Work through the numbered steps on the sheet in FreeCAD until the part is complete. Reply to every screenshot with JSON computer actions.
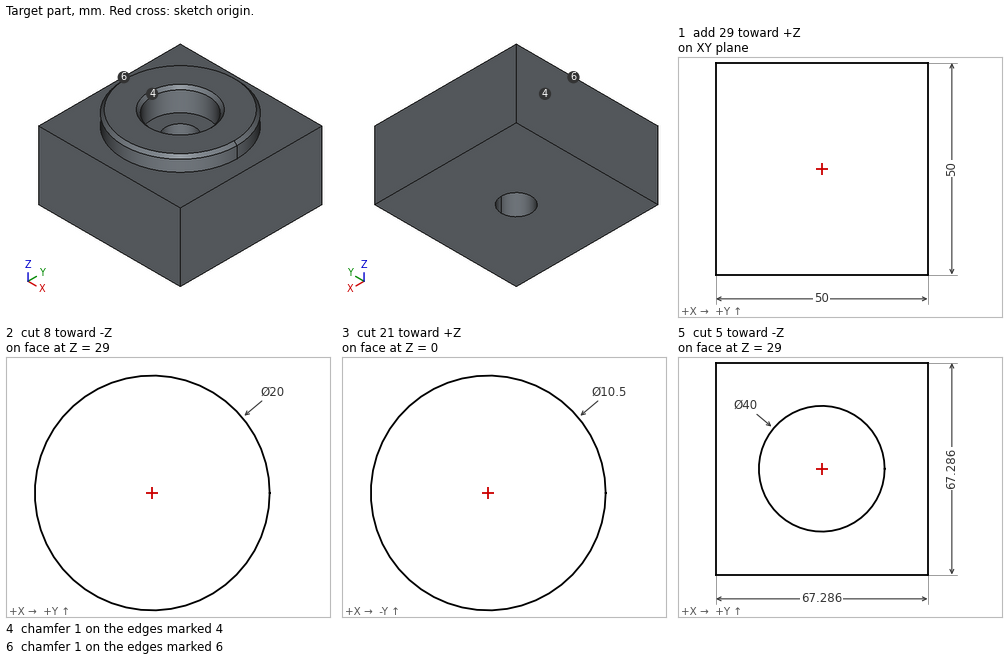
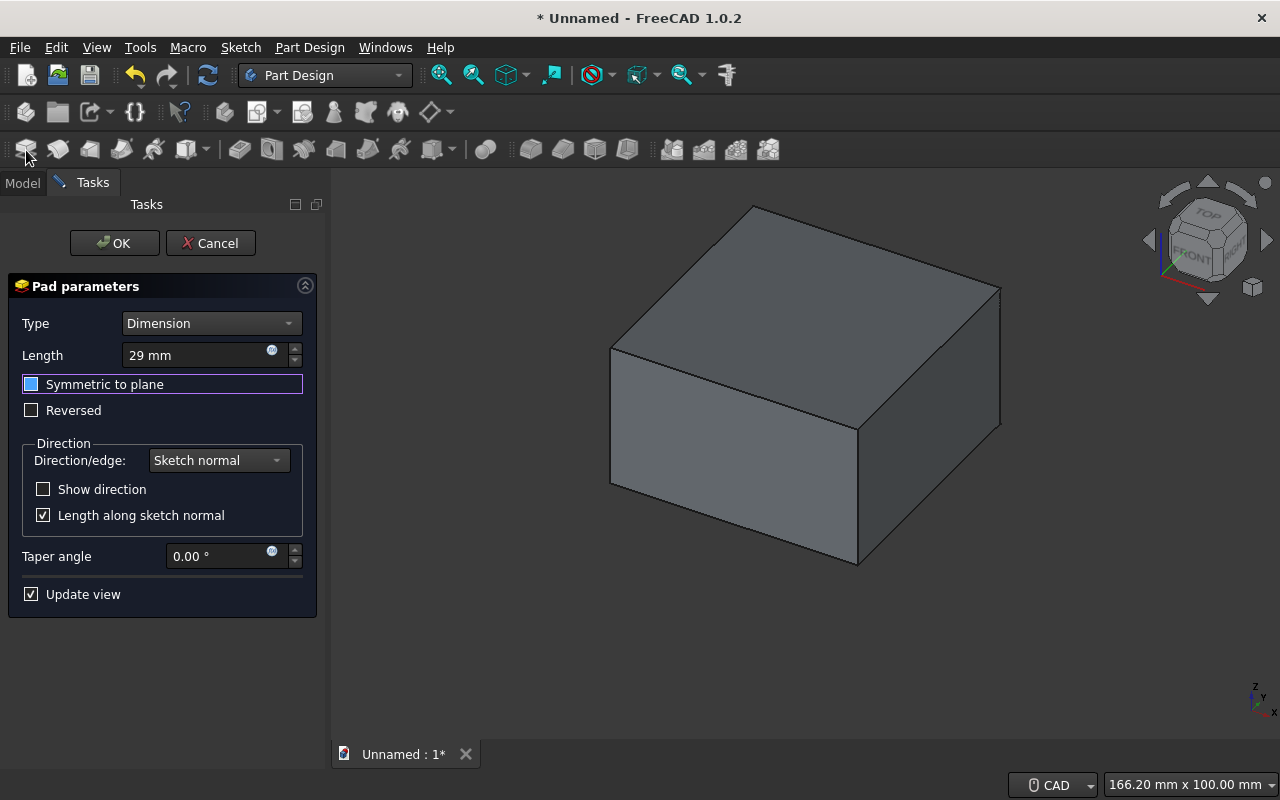
{"action": "left_click", "coordinate": [115, 243]}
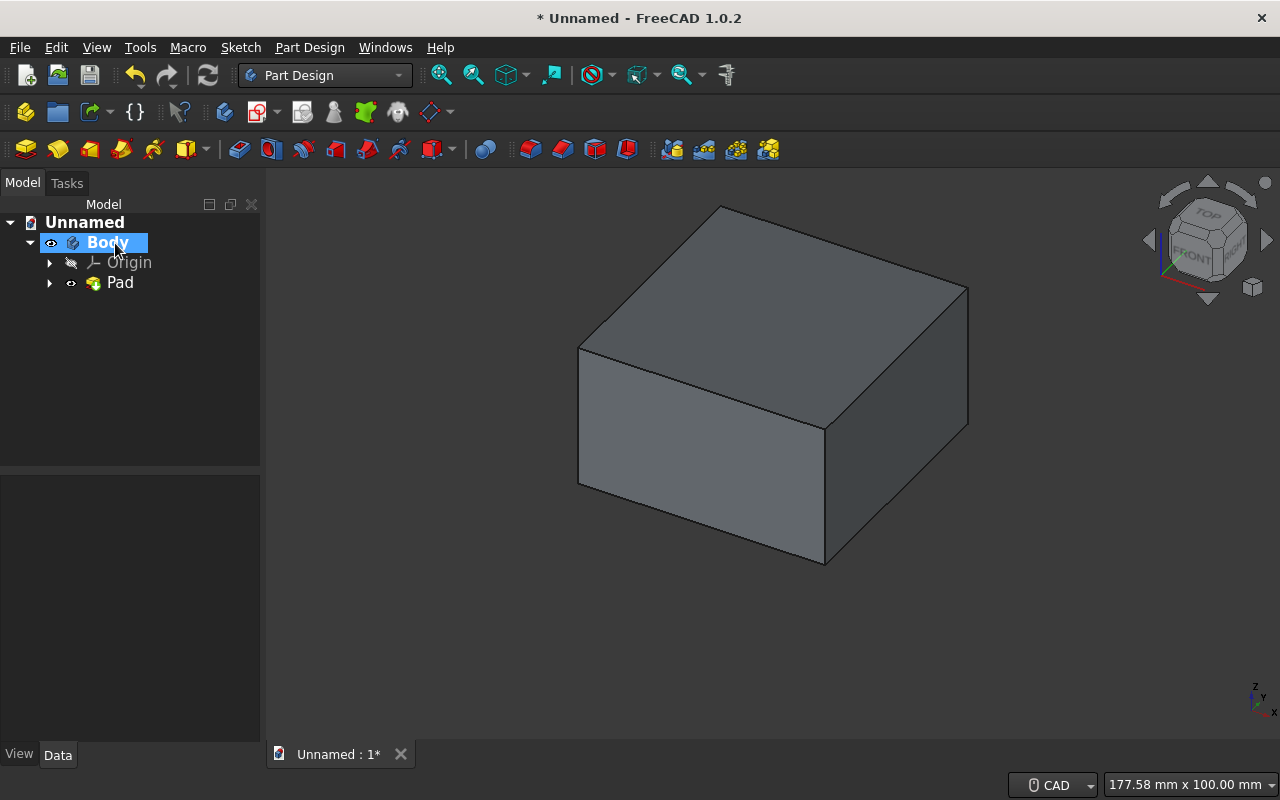
{"action": "left_click", "coordinate": [773, 317]}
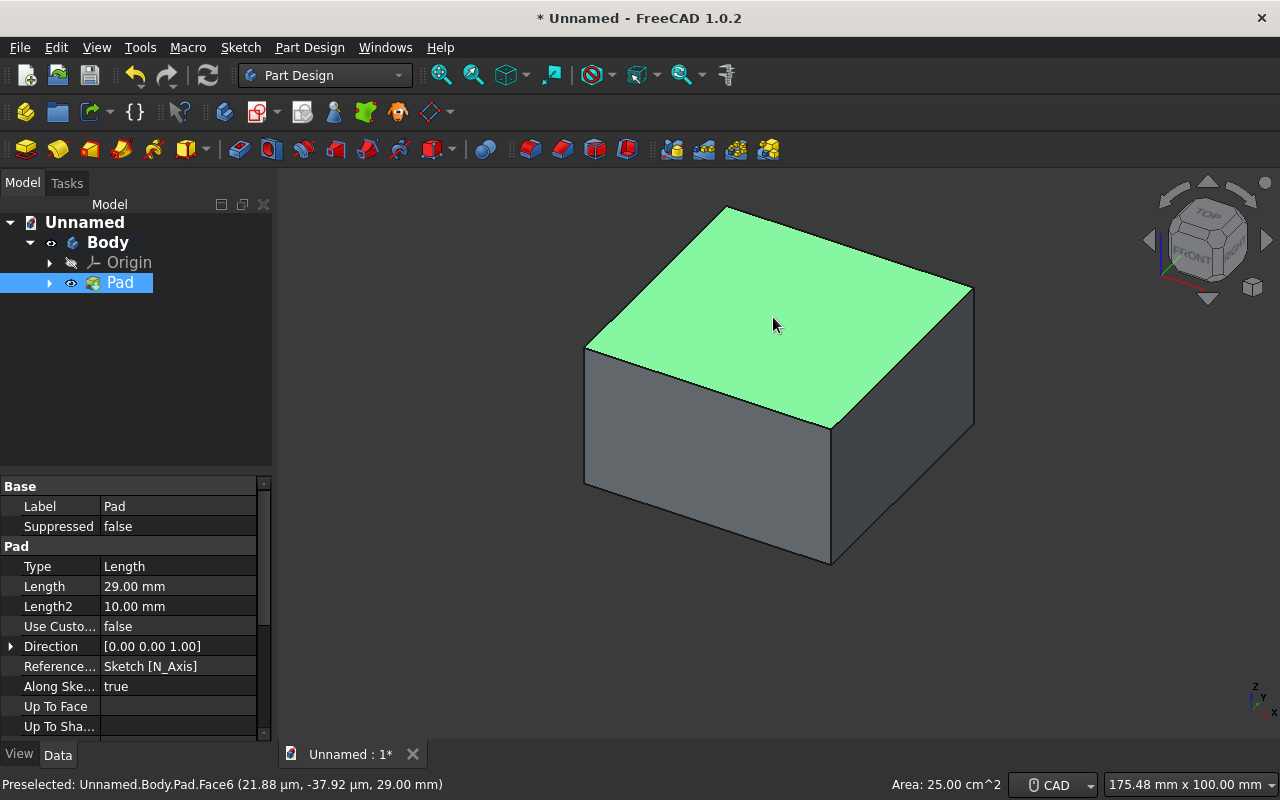
{"action": "left_click", "coordinate": [258, 112]}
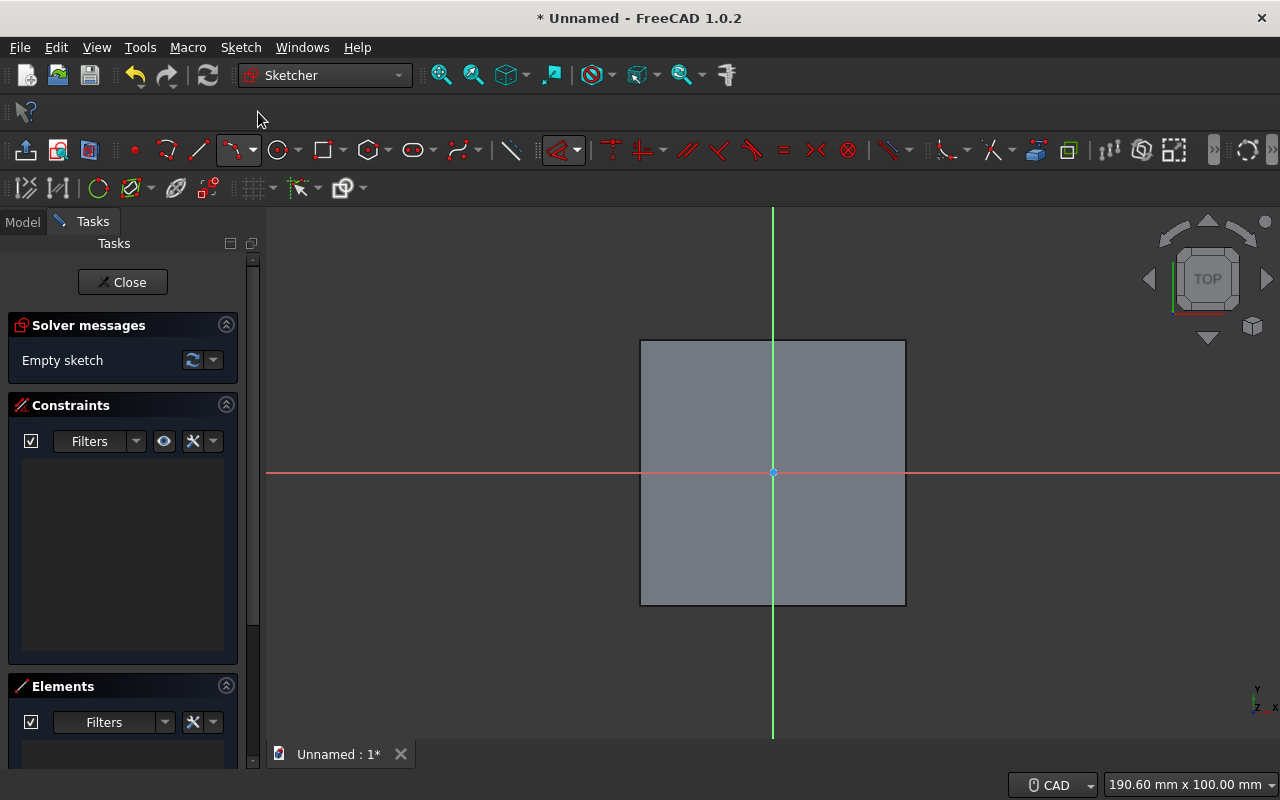
{"action": "scroll", "coordinate": [803, 473], "scroll_direction": "up", "scroll_amount": 6}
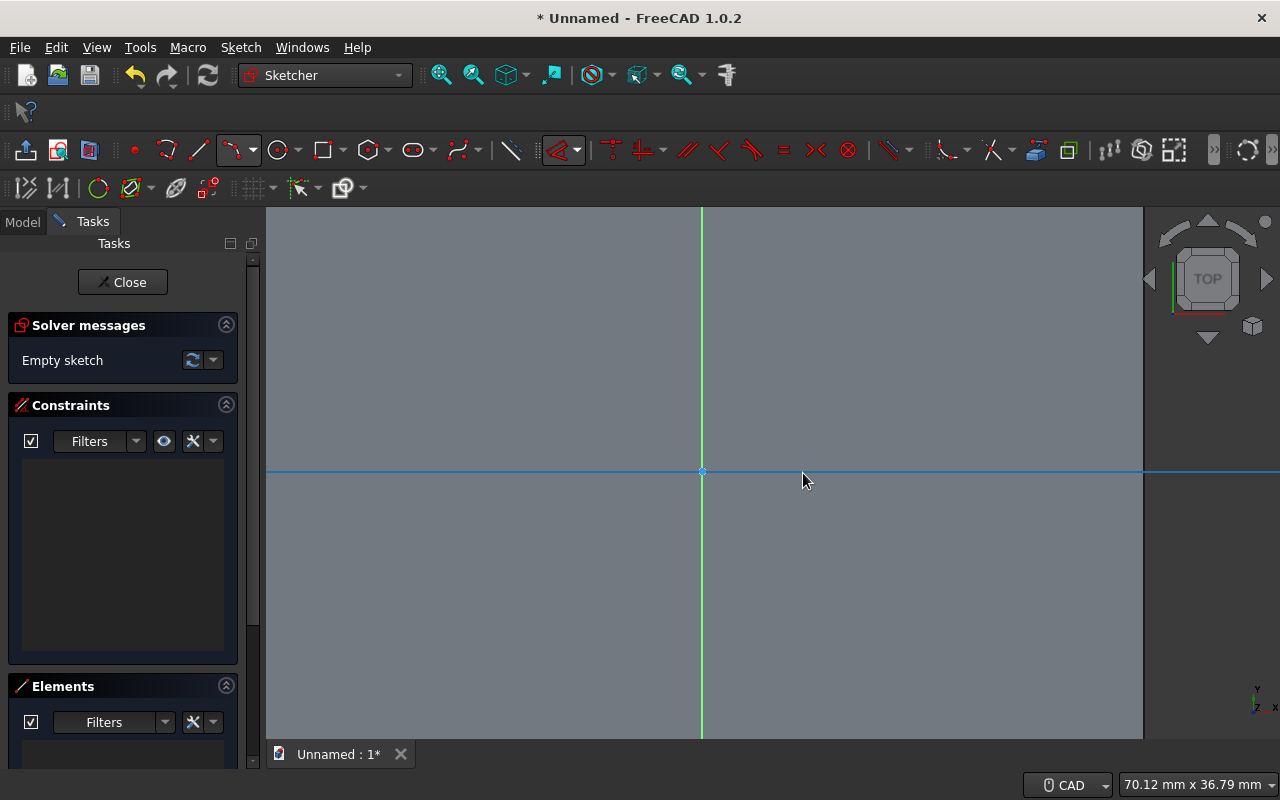
{"action": "left_click", "coordinate": [278, 150]}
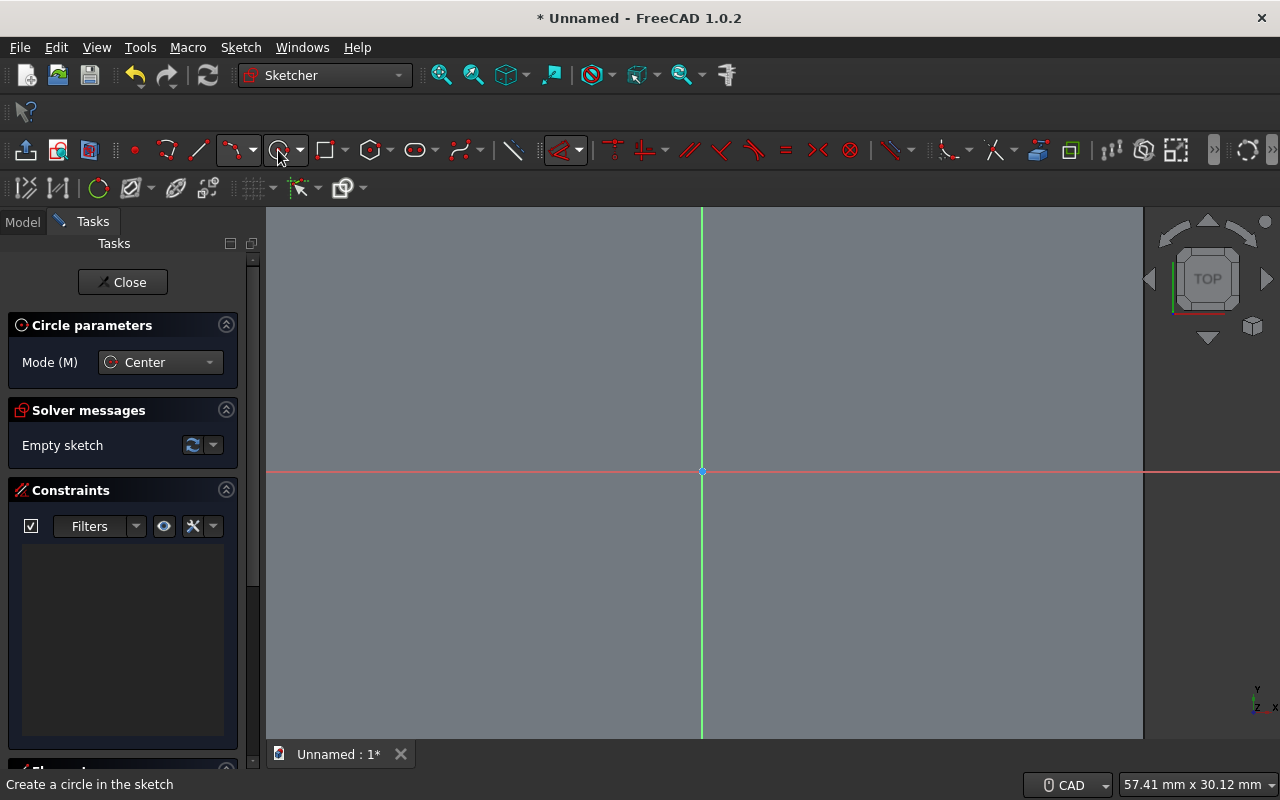
{"action": "left_click", "coordinate": [702, 472]}
{"action": "mouse_move", "coordinate": [827, 347]}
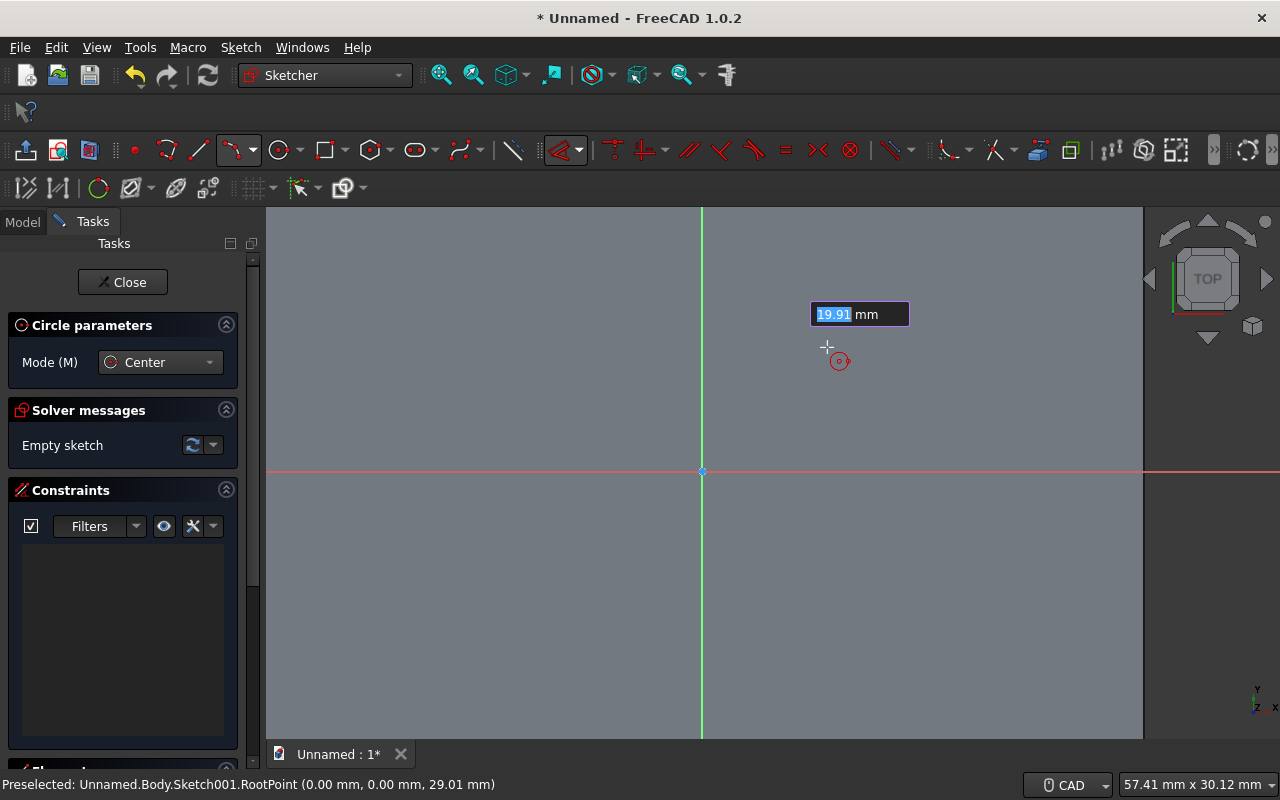
{"action": "type", "text": "20"}
{"action": "key", "text": "Return"}
{"action": "key", "text": "Escape"}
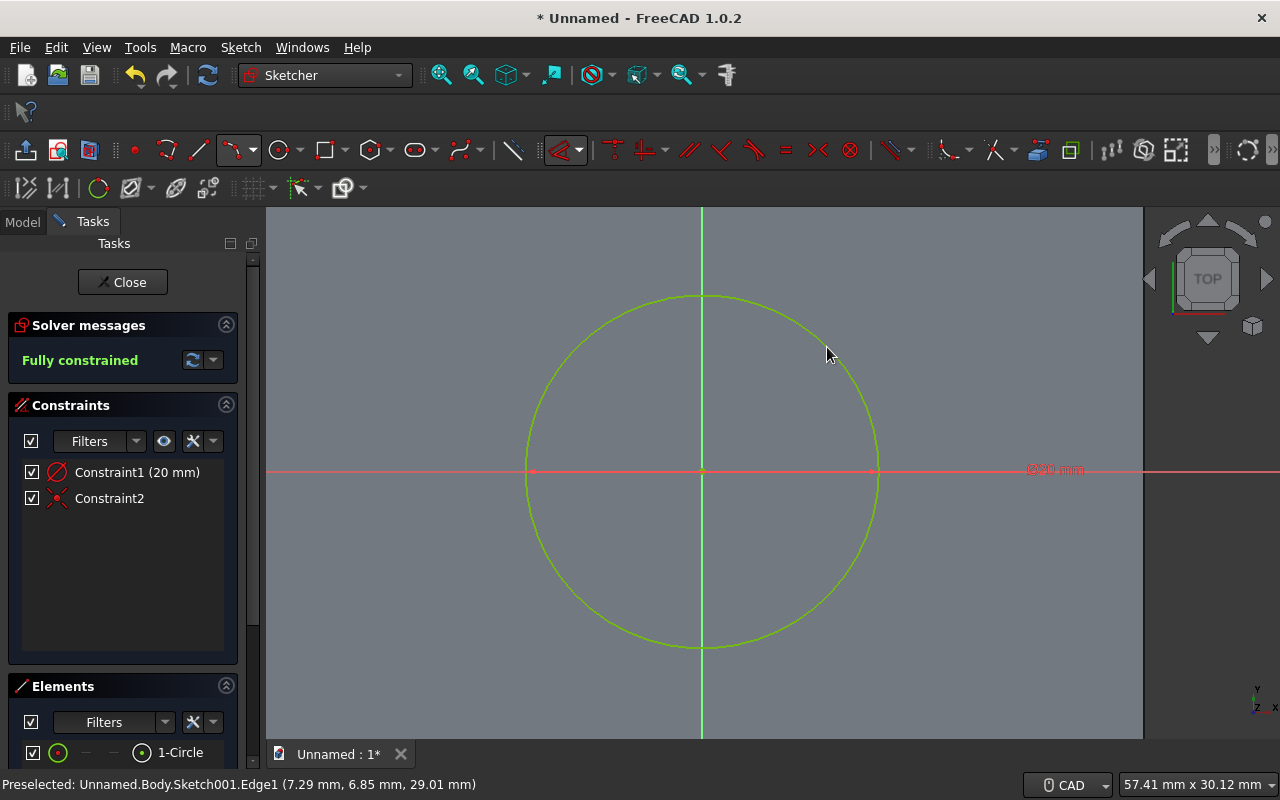
{"action": "left_click", "coordinate": [123, 282]}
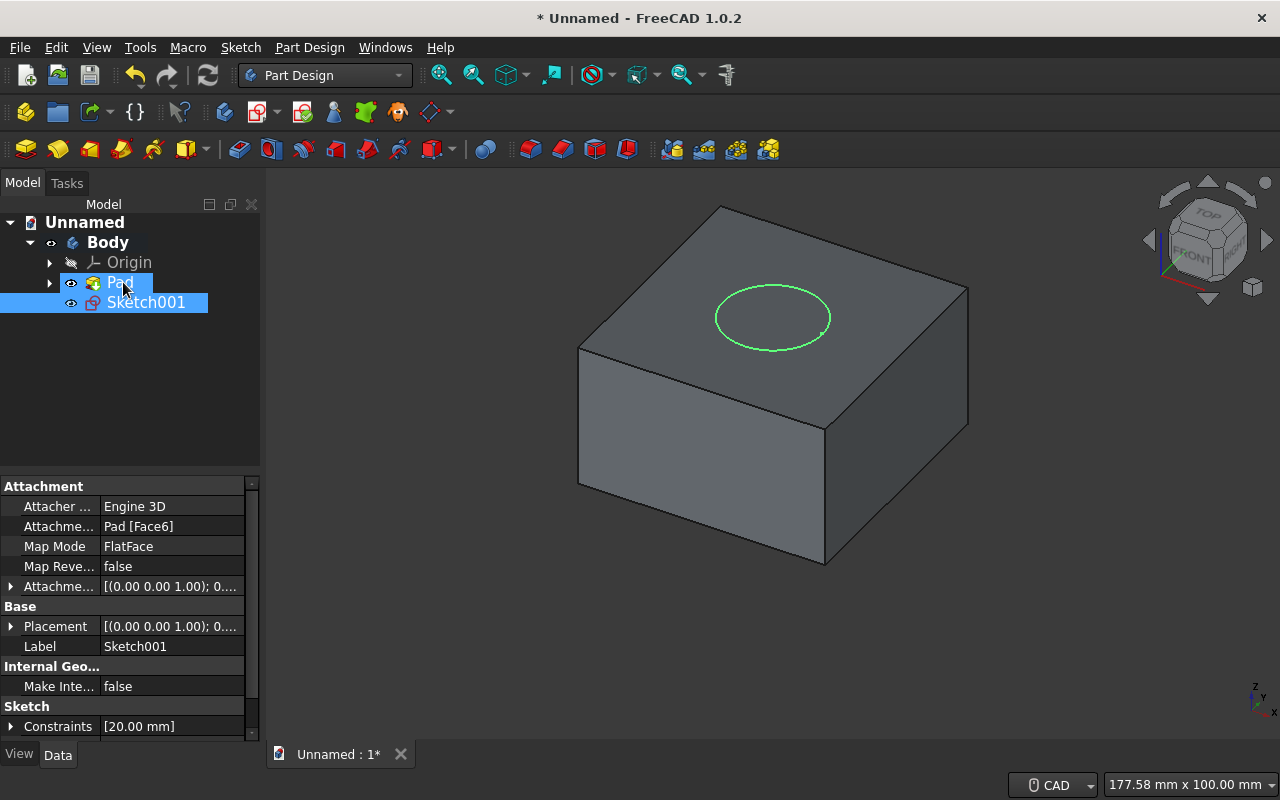
{"action": "left_click", "coordinate": [240, 150]}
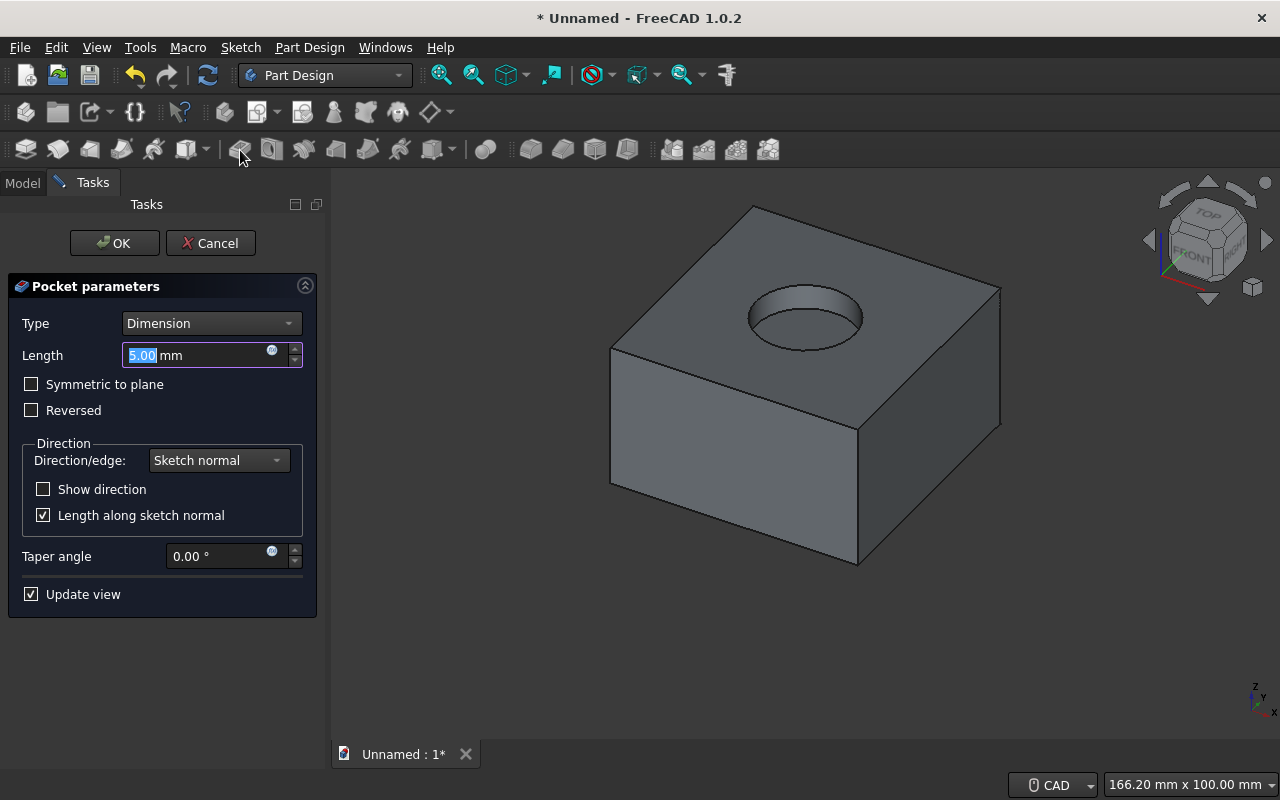
{"action": "type", "text": "8"}
{"action": "key", "text": "Tab"}